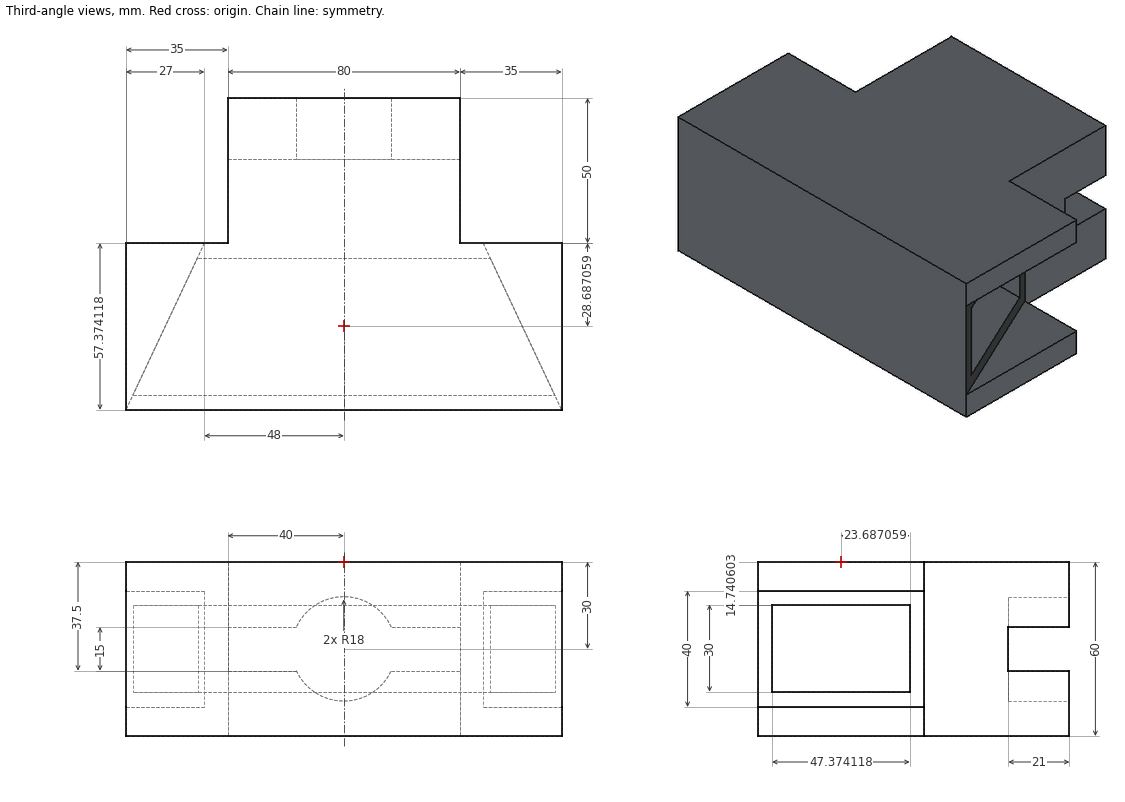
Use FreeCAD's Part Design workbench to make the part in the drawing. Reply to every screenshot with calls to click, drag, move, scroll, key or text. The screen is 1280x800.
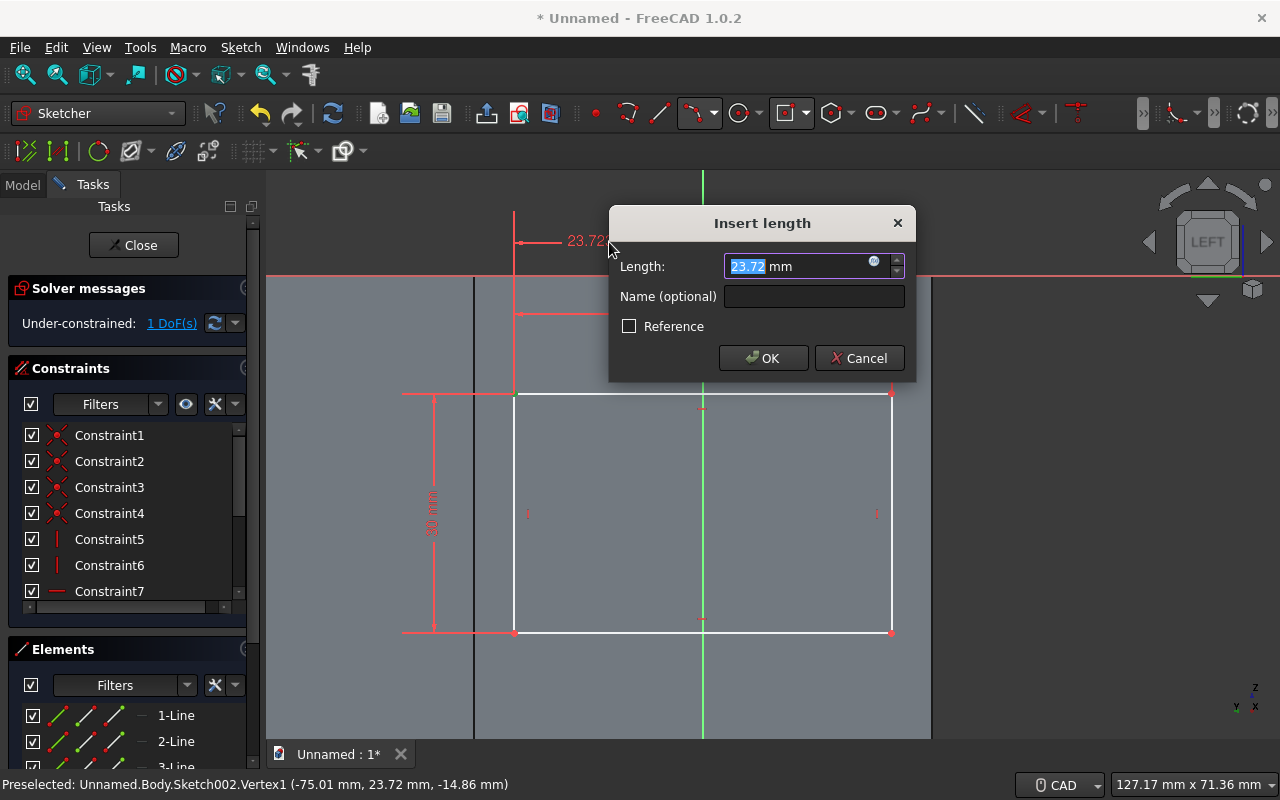
text(23.687059)
key(Return)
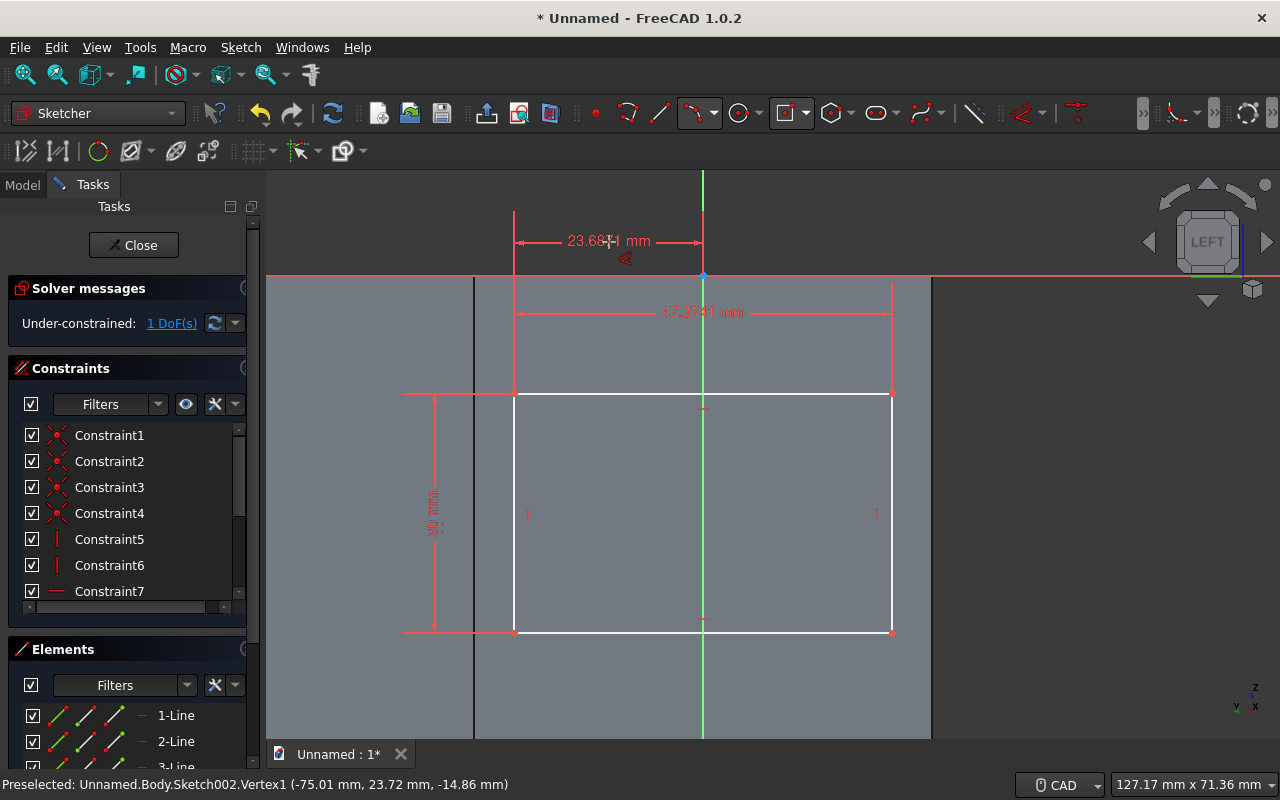
click(514, 394)
click(480, 335)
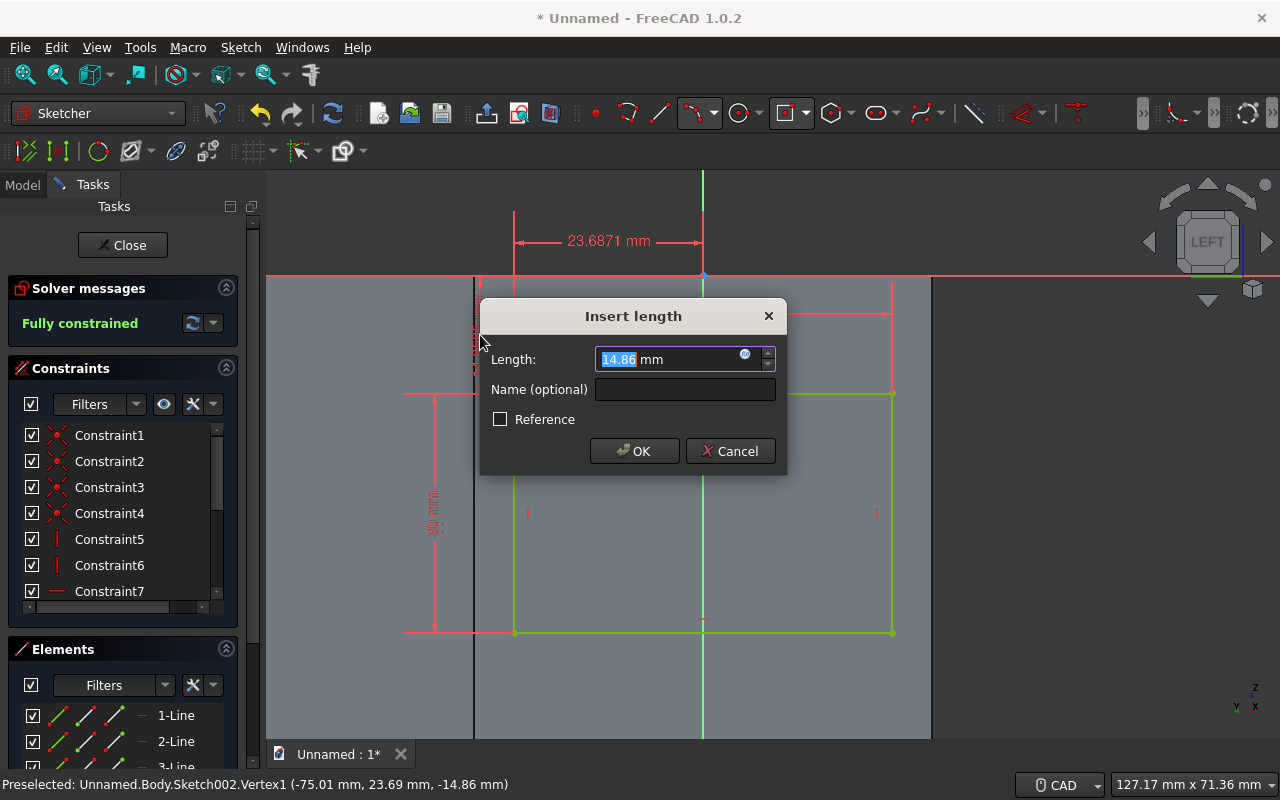
text(14.740603)
key(Return)
key(Escape)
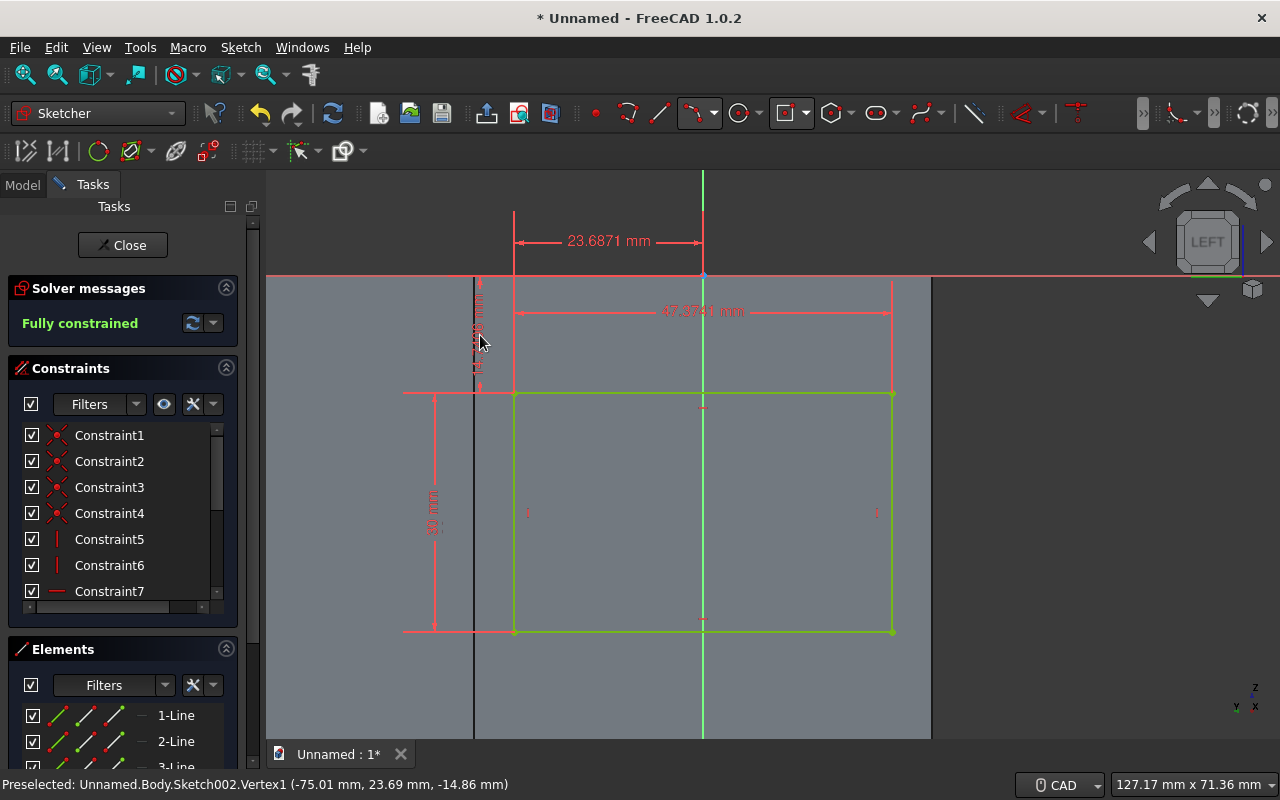
click(123, 245)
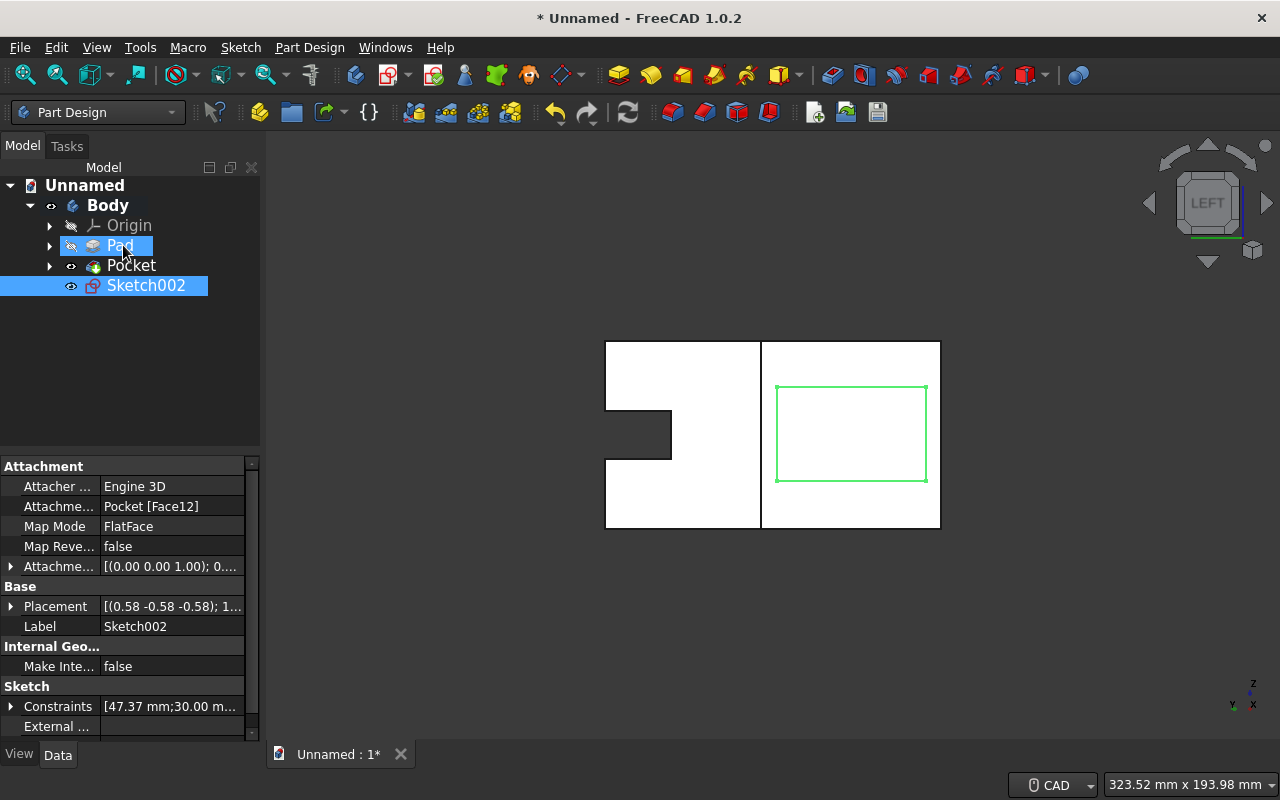
click(834, 76)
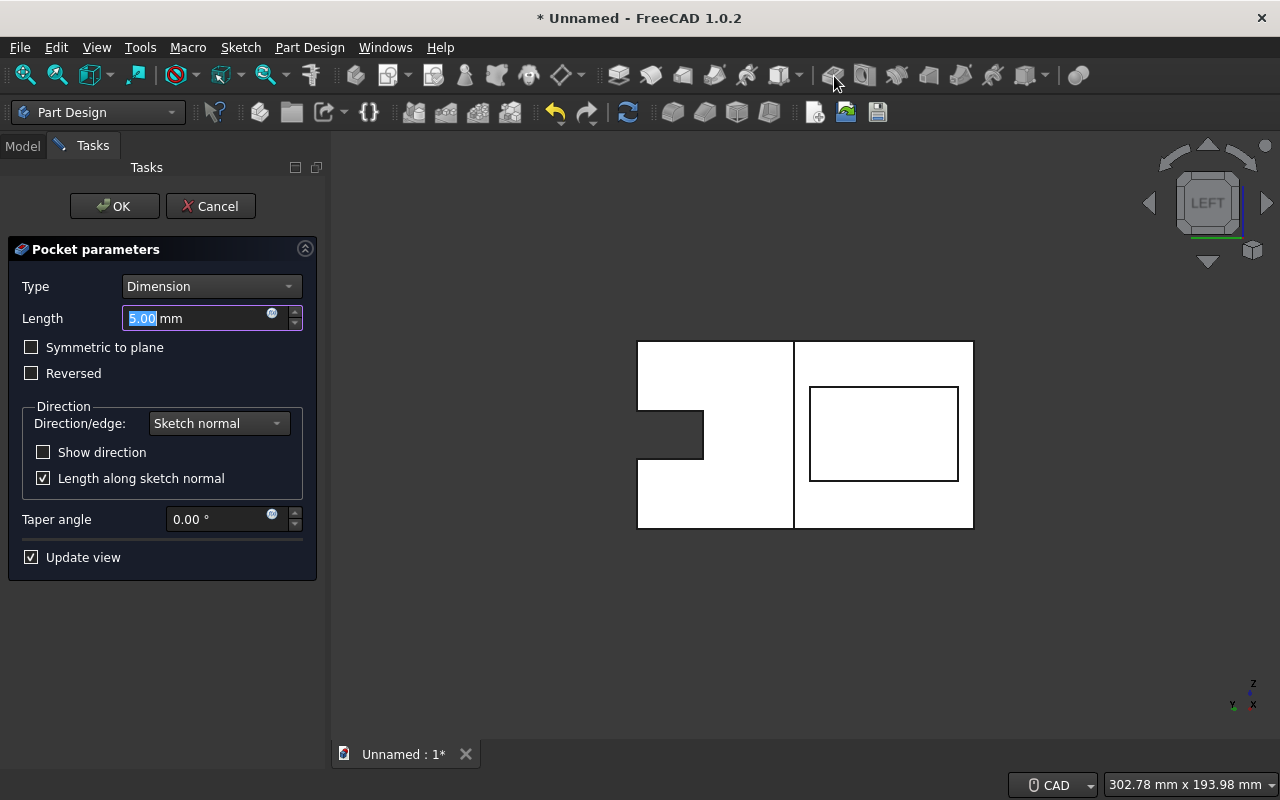
click(212, 286)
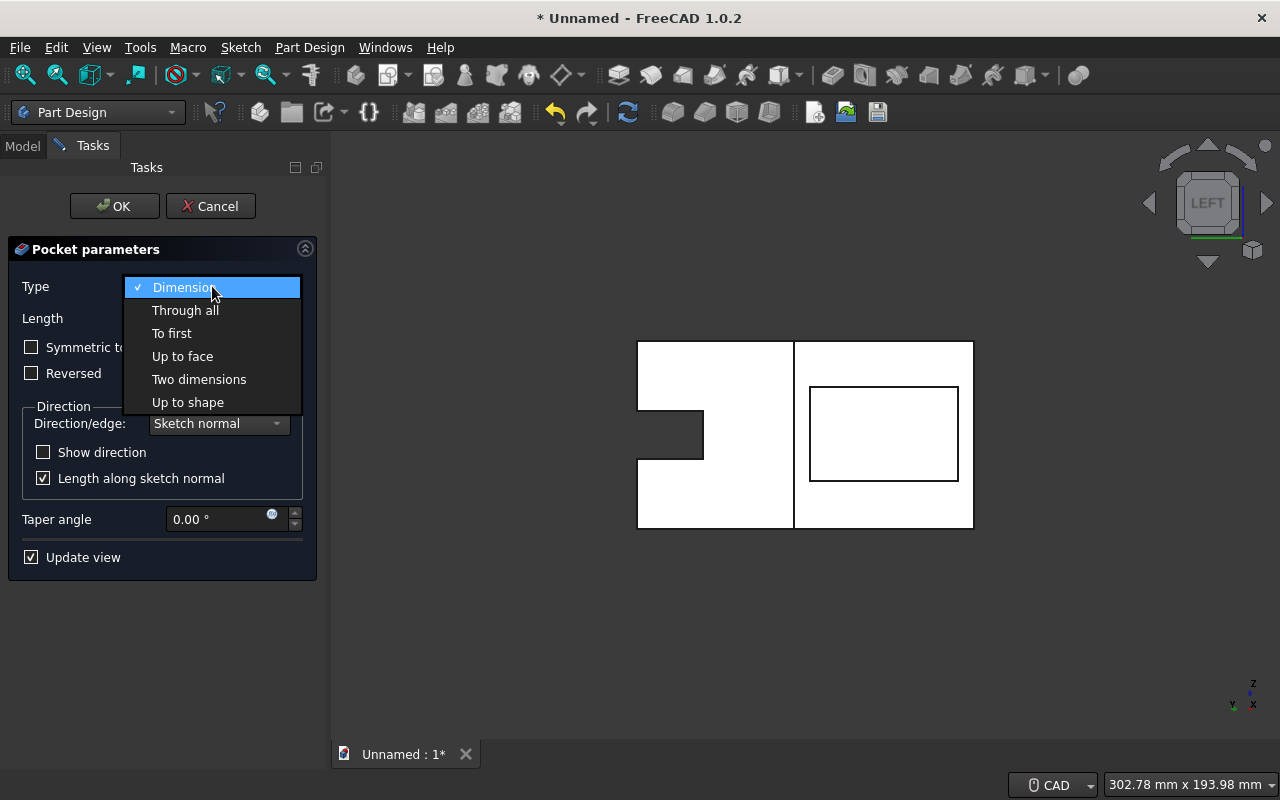
click(212, 310)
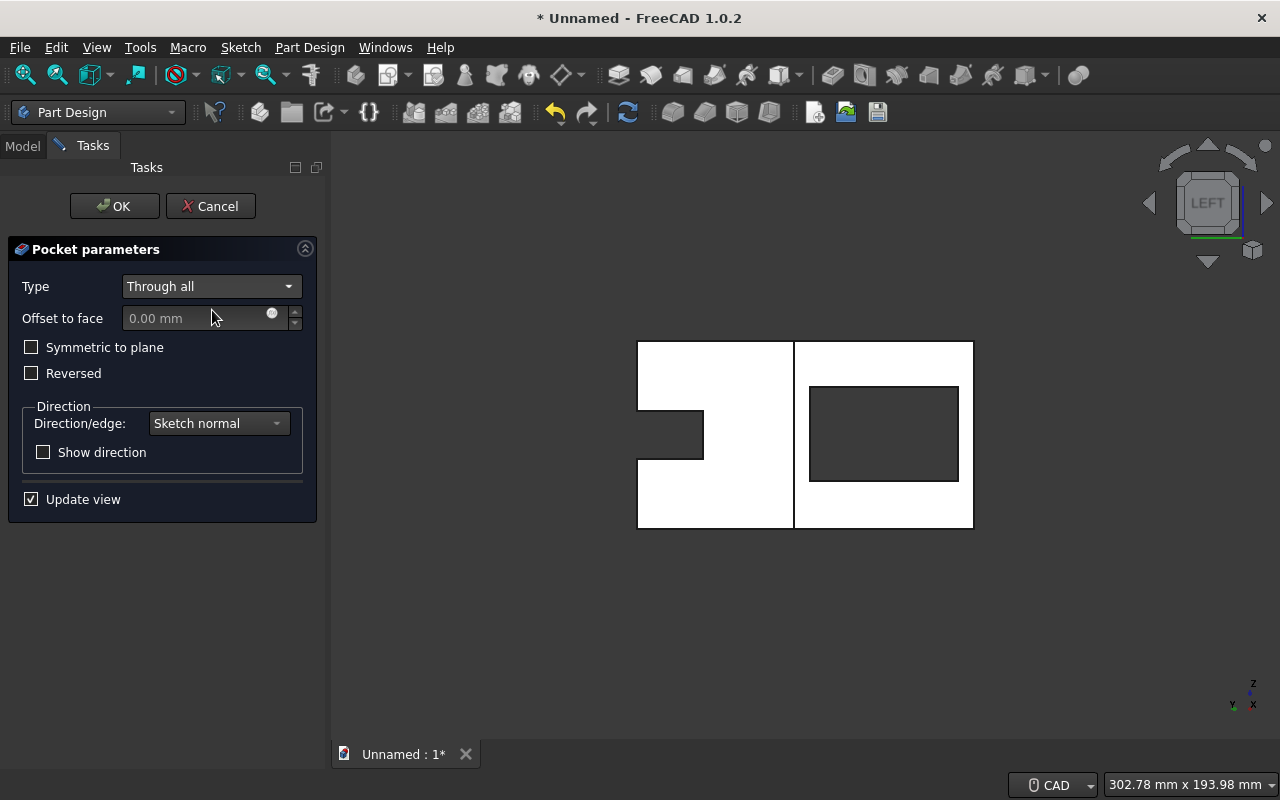
click(115, 206)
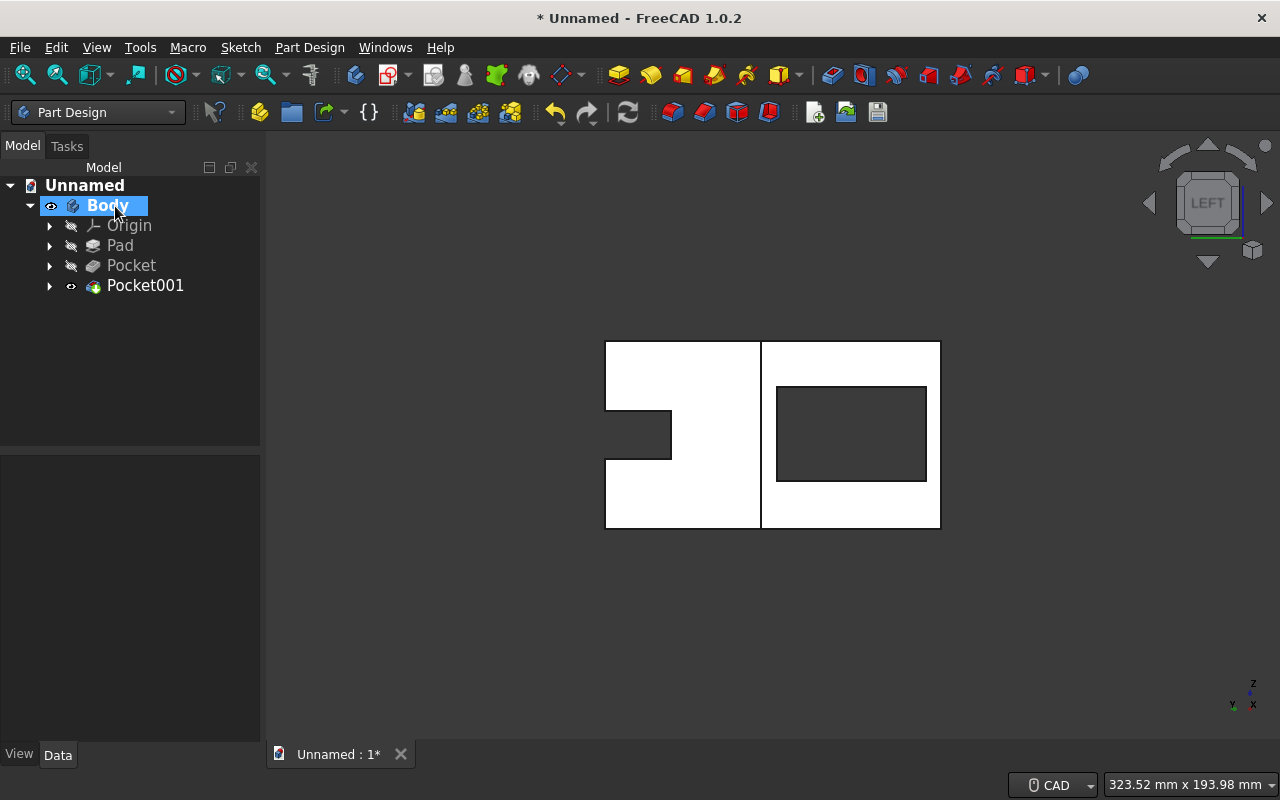
key(v)
key(f)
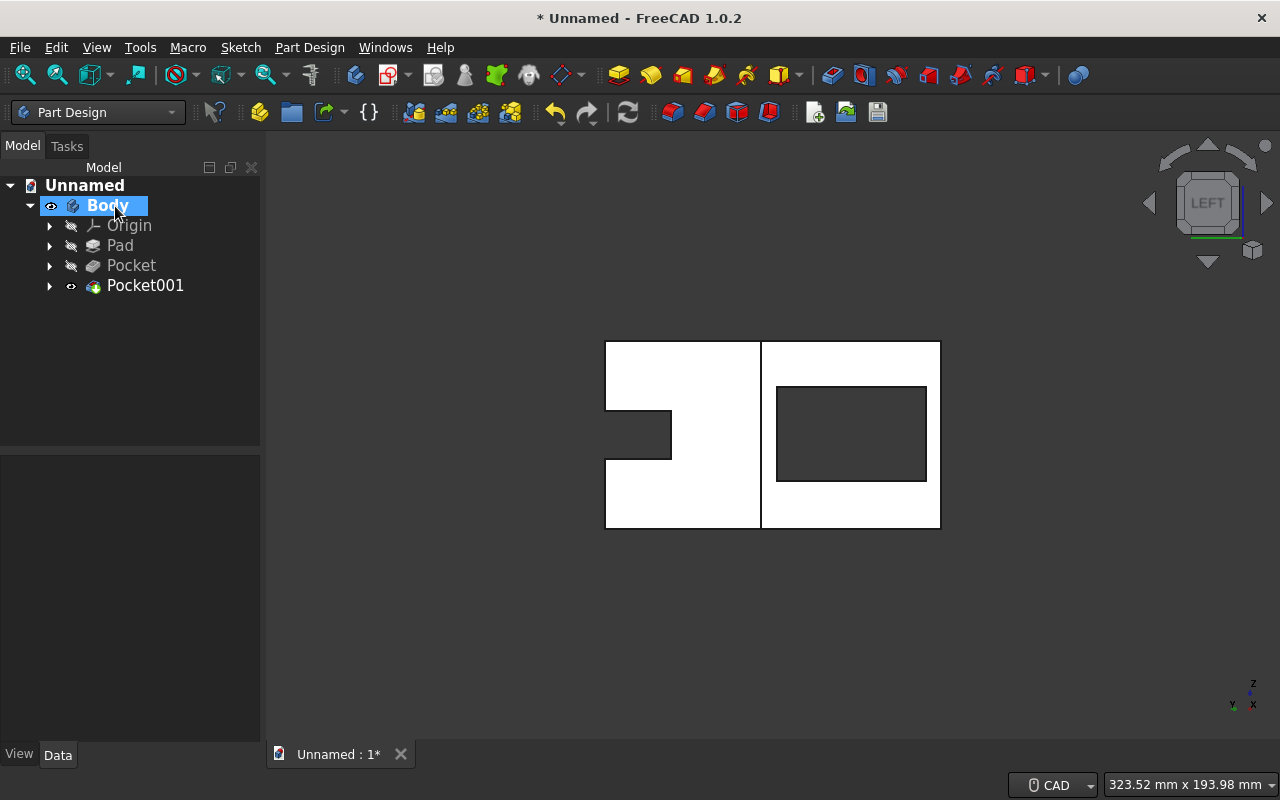
click(50, 226)